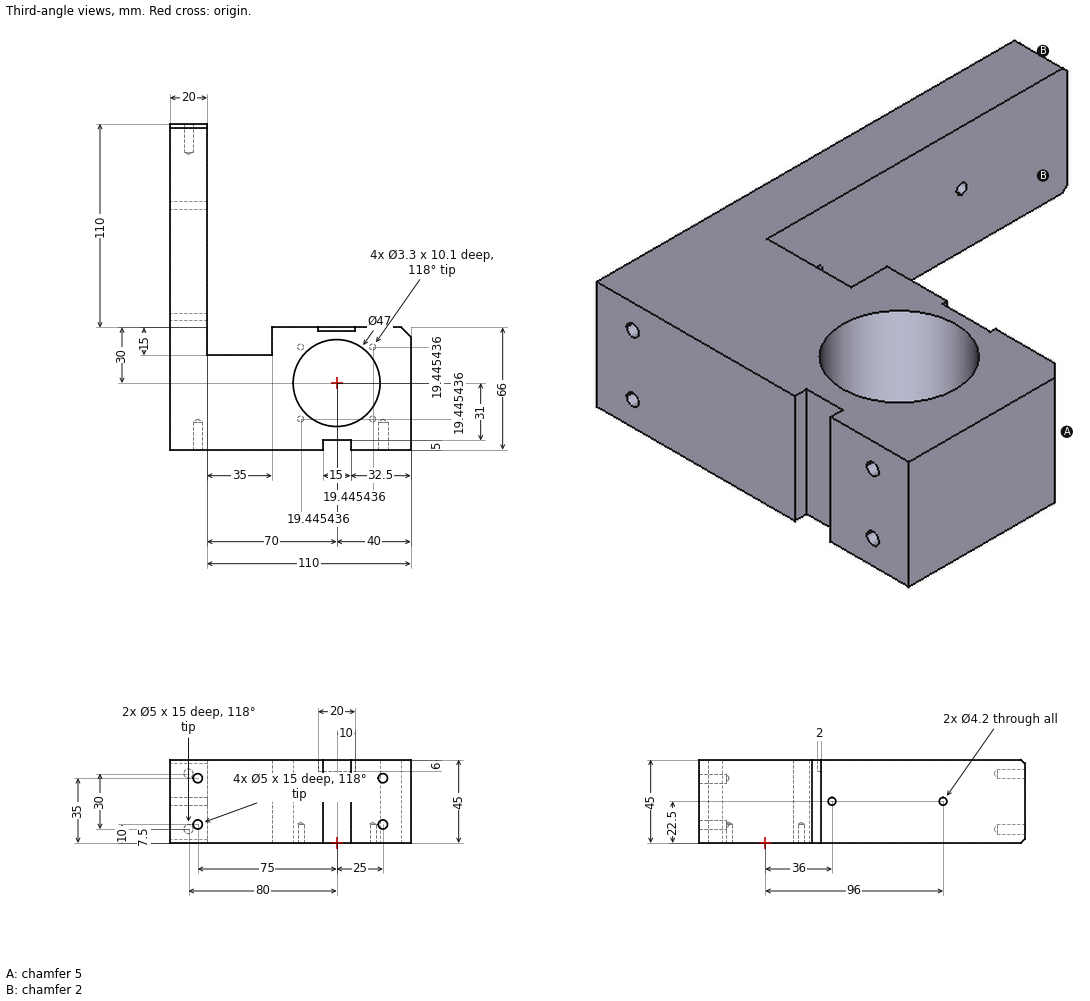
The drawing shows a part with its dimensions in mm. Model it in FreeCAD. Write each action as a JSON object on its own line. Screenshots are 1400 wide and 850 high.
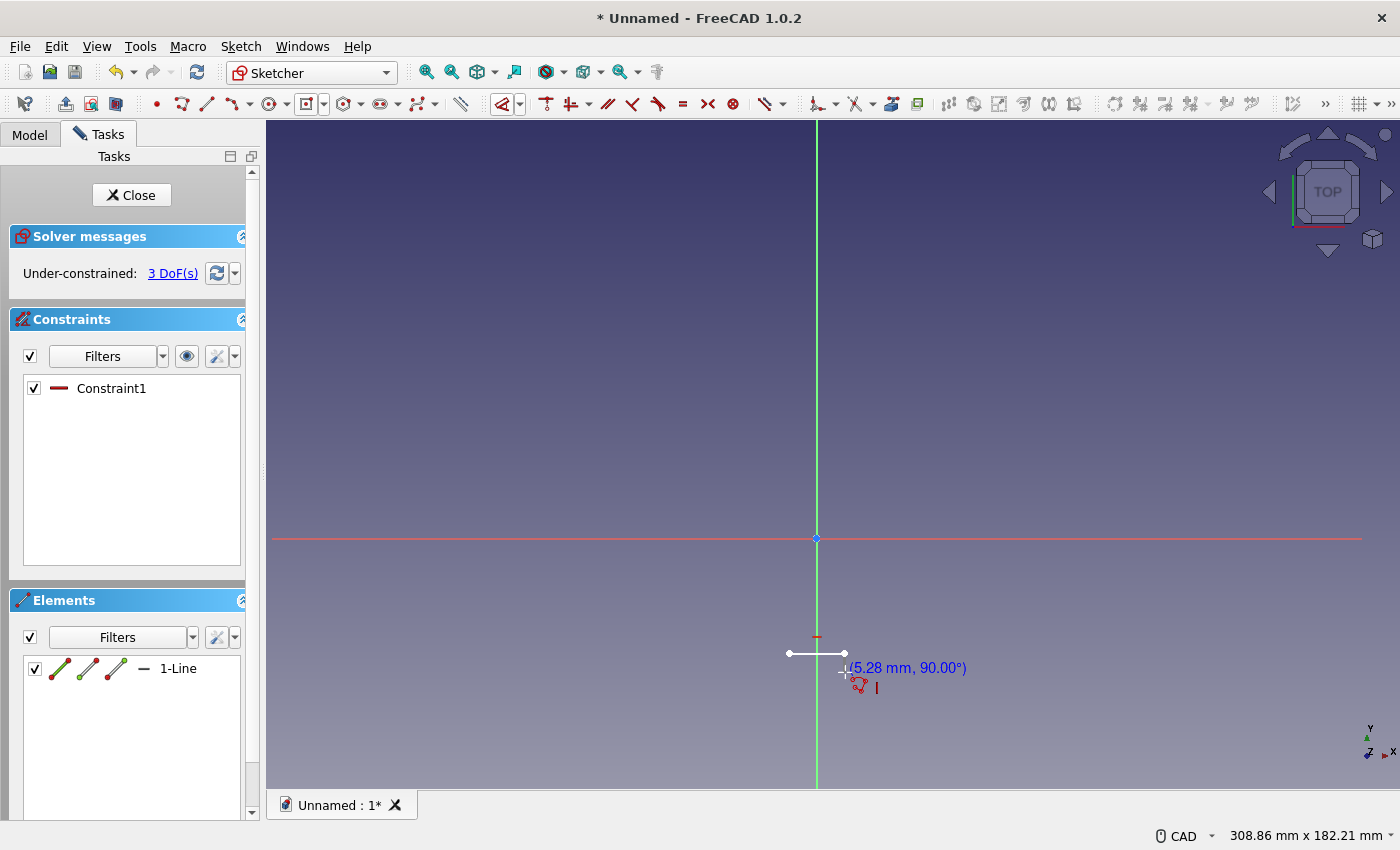
{"action": "left_click", "coordinate": [845, 671]}
{"action": "left_click", "coordinate": [964, 671]}
{"action": "left_click", "coordinate": [964, 429]}
{"action": "left_click", "coordinate": [560, 429]}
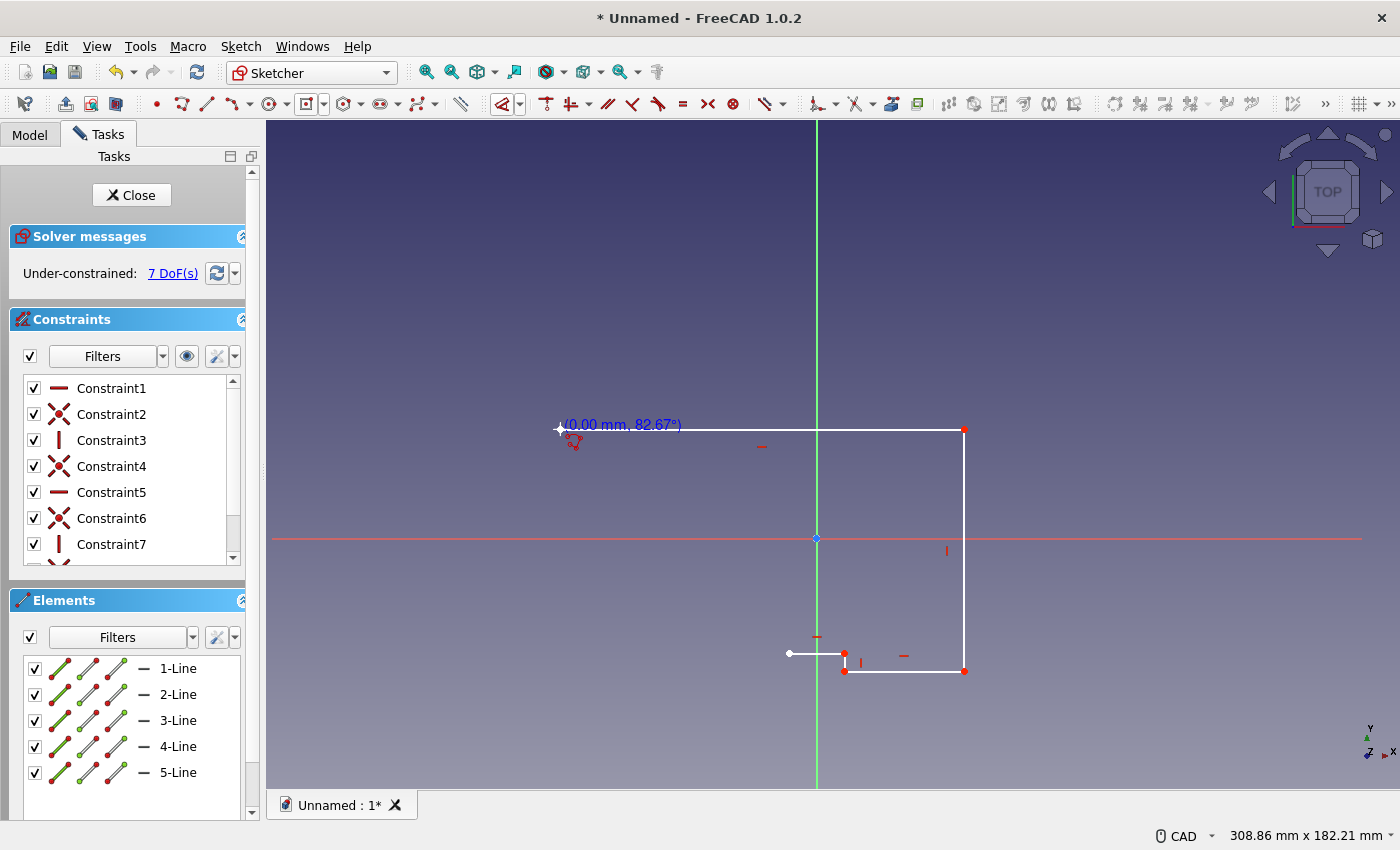
{"action": "scroll", "coordinate": [845, 671], "scroll_direction": "down", "scroll_amount": 2}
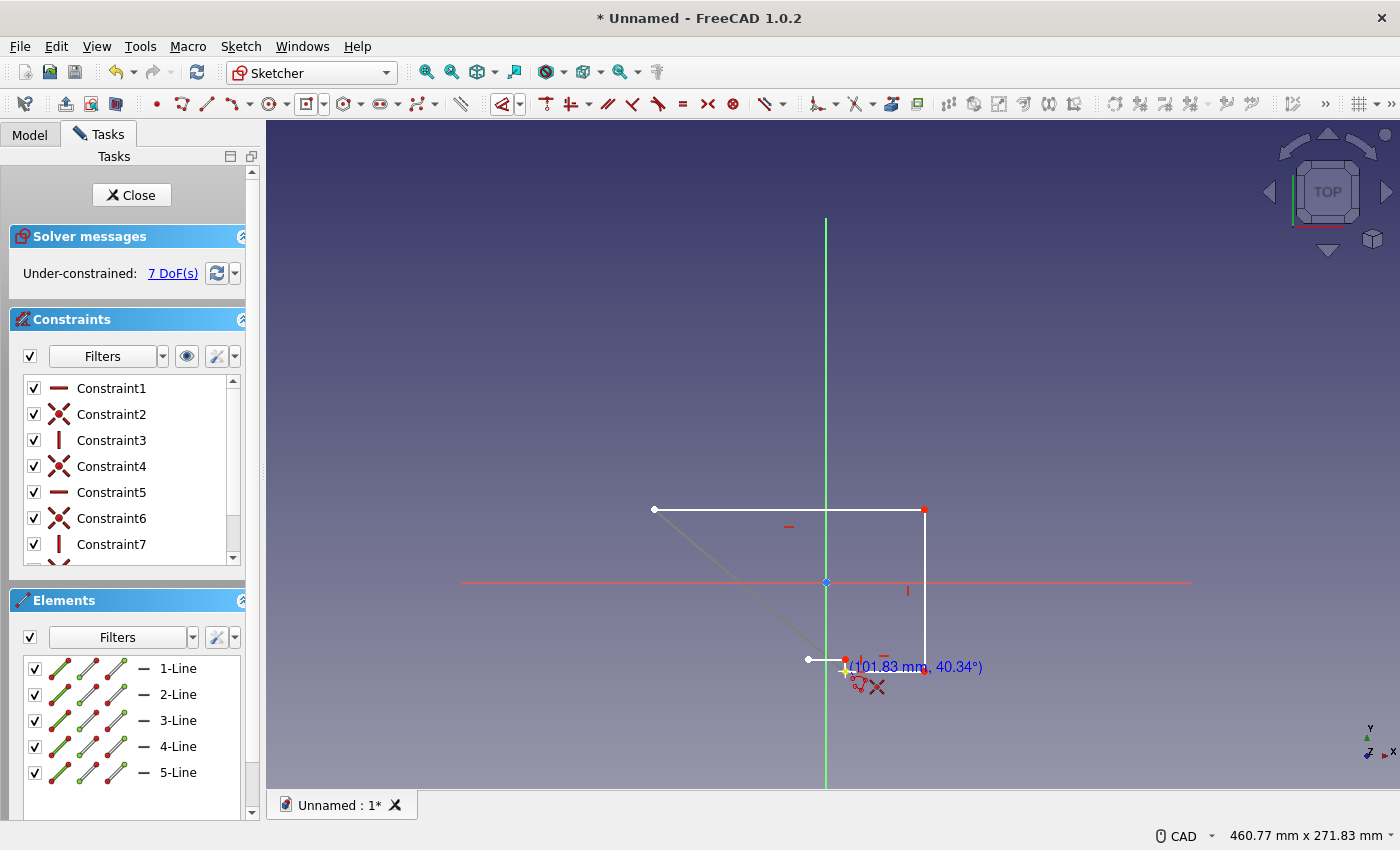
{"action": "left_click", "coordinate": [654, 238]}
{"action": "left_click", "coordinate": [605, 238]}
{"action": "left_click", "coordinate": [605, 671]}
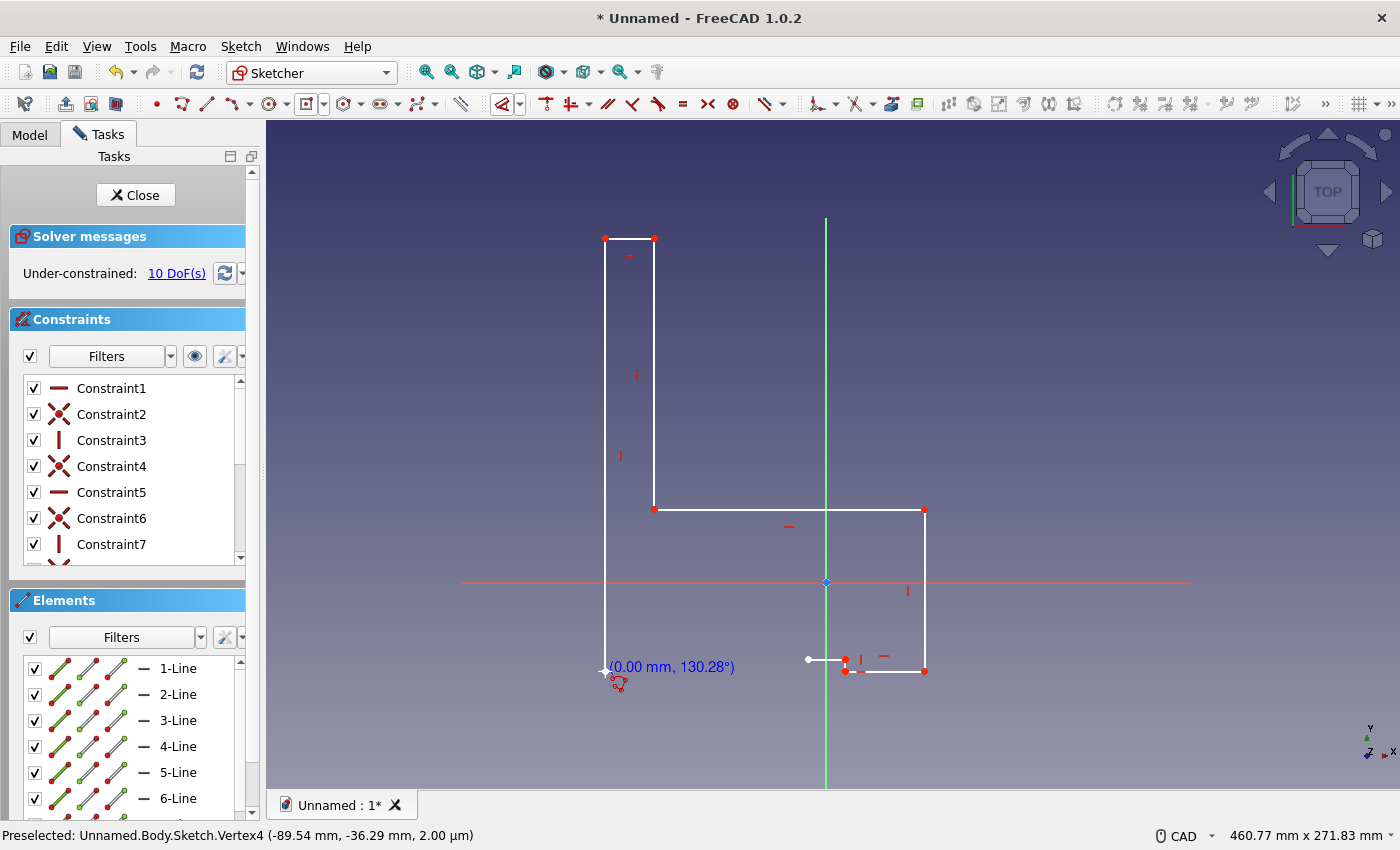
{"action": "scroll", "coordinate": [808, 671], "scroll_direction": "up", "scroll_amount": 2}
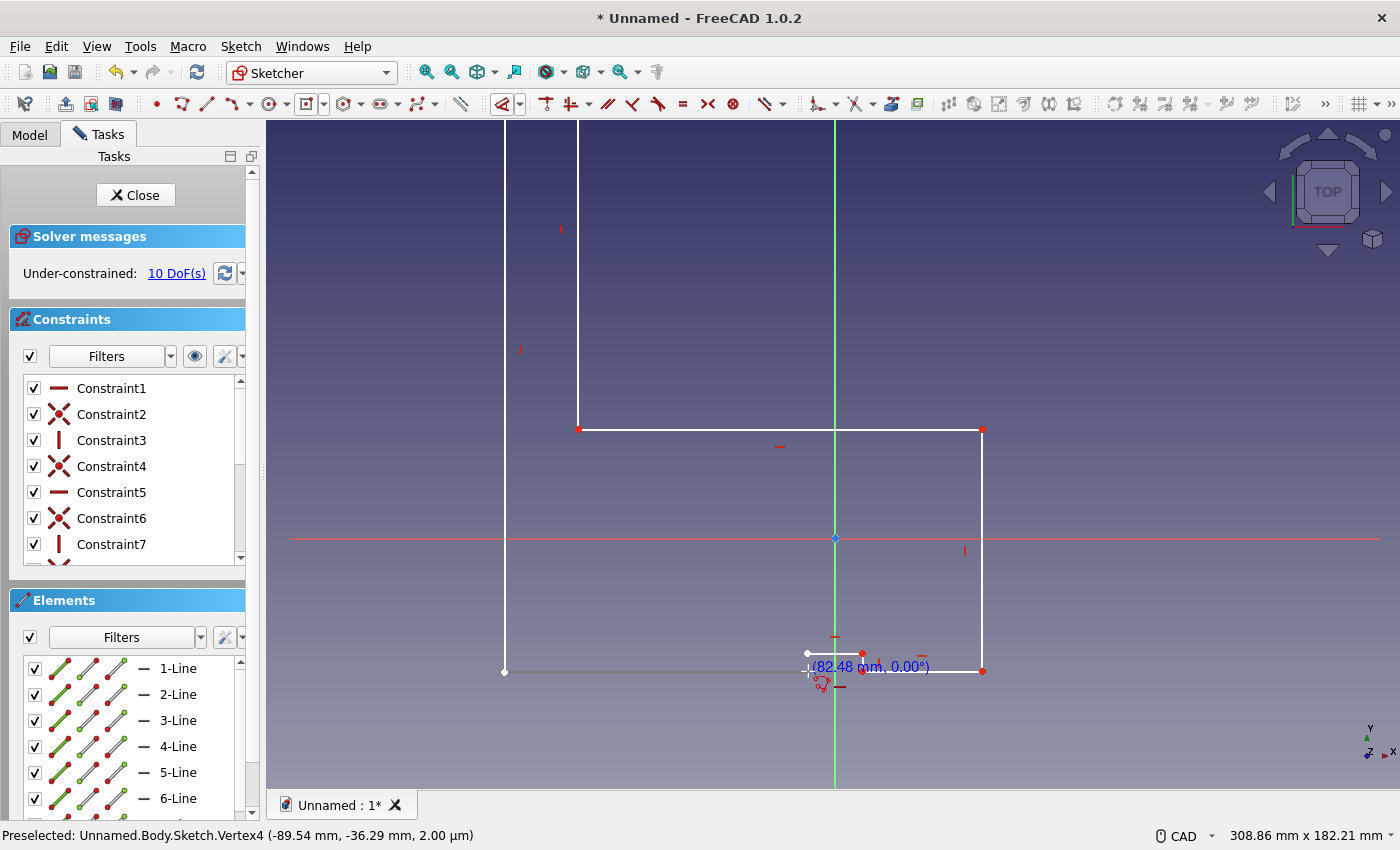
{"action": "left_click", "coordinate": [808, 671]}
{"action": "left_click", "coordinate": [808, 654]}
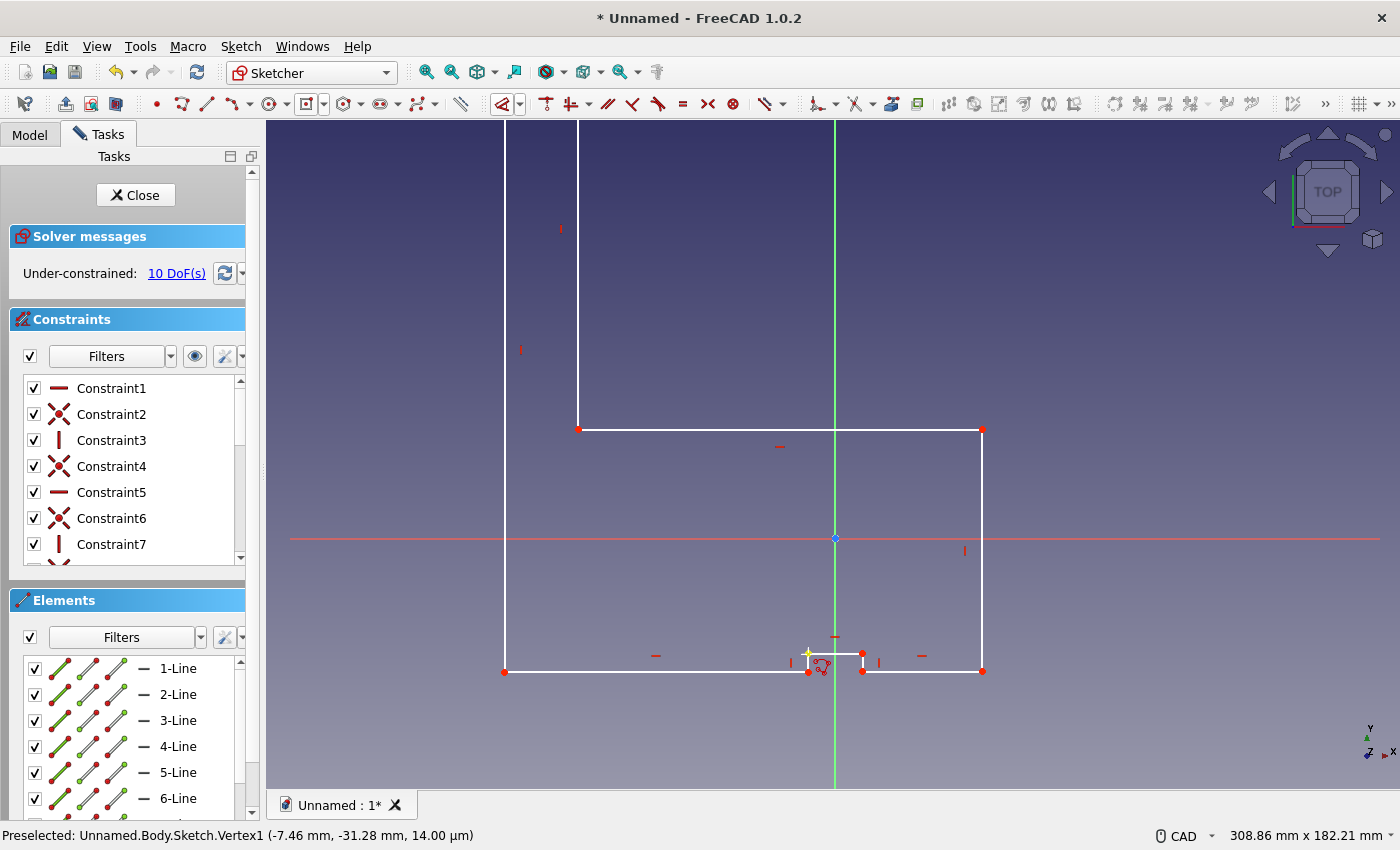
{"action": "left_click", "coordinate": [268, 104]}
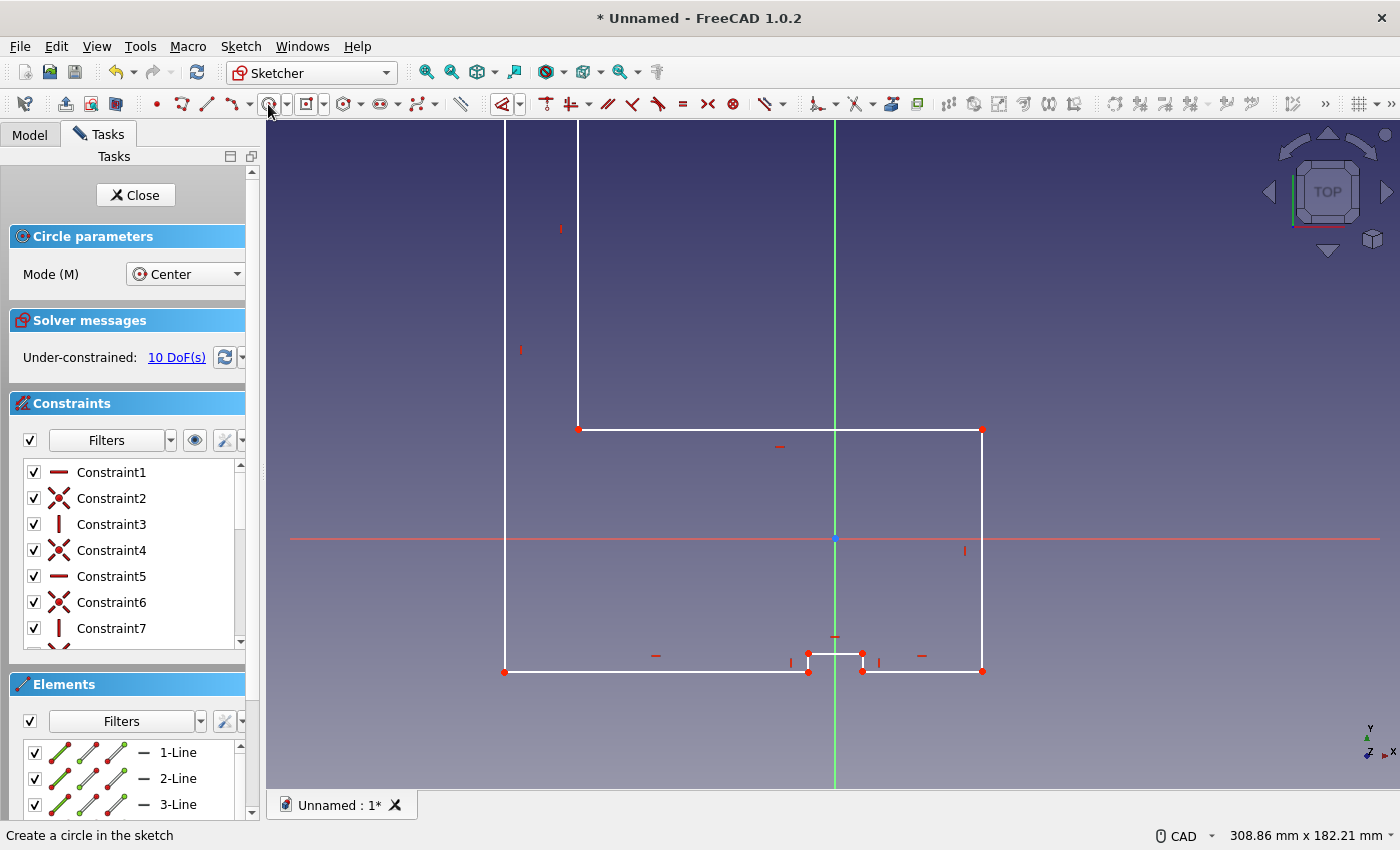
{"action": "left_click", "coordinate": [835, 539]}
{"action": "left_click", "coordinate": [896, 478]}
{"action": "key", "text": "Escape"}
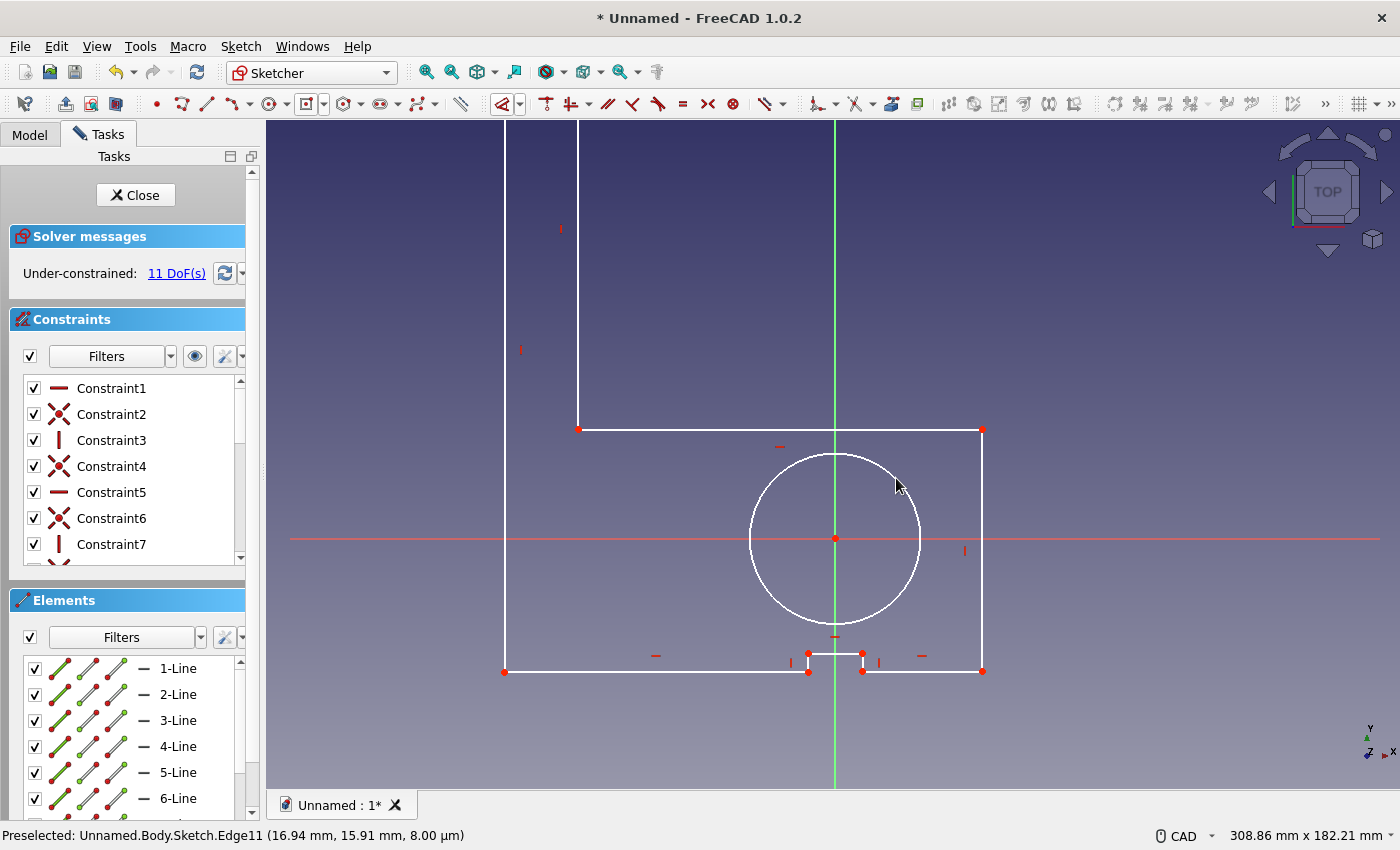
{"action": "key", "text": "d"}